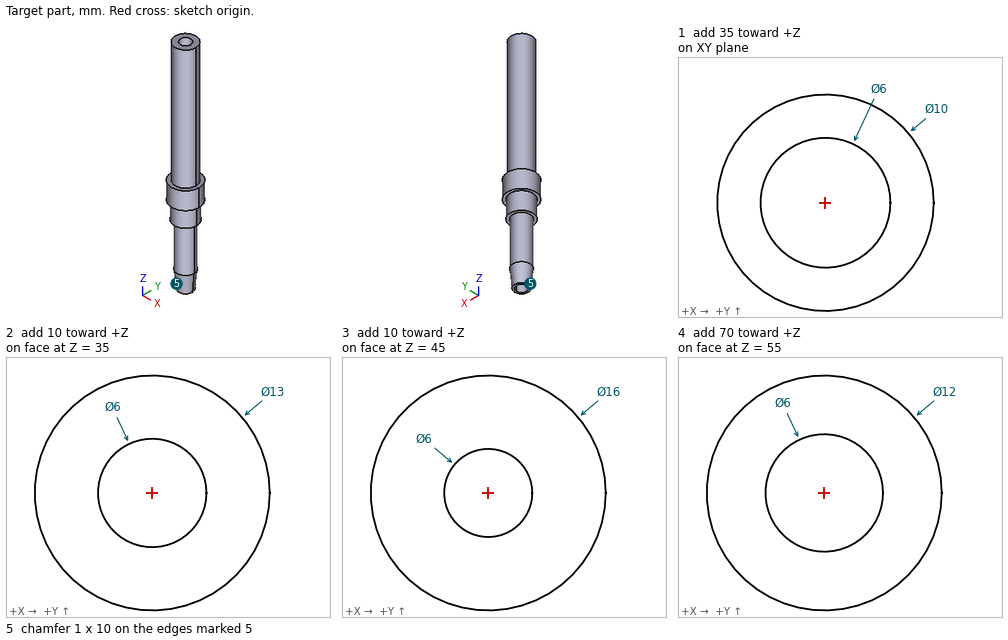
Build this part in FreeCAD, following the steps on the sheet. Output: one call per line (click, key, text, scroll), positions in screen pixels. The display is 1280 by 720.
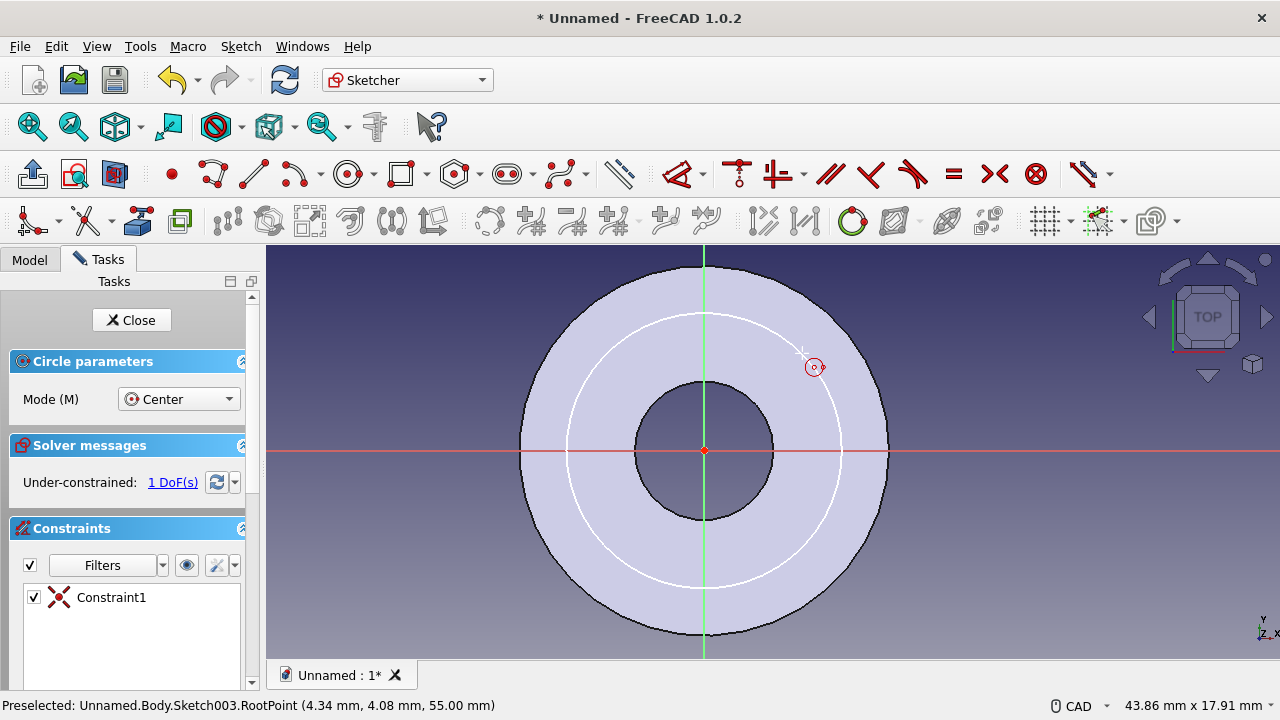
click(704, 451)
click(753, 402)
key(Escape)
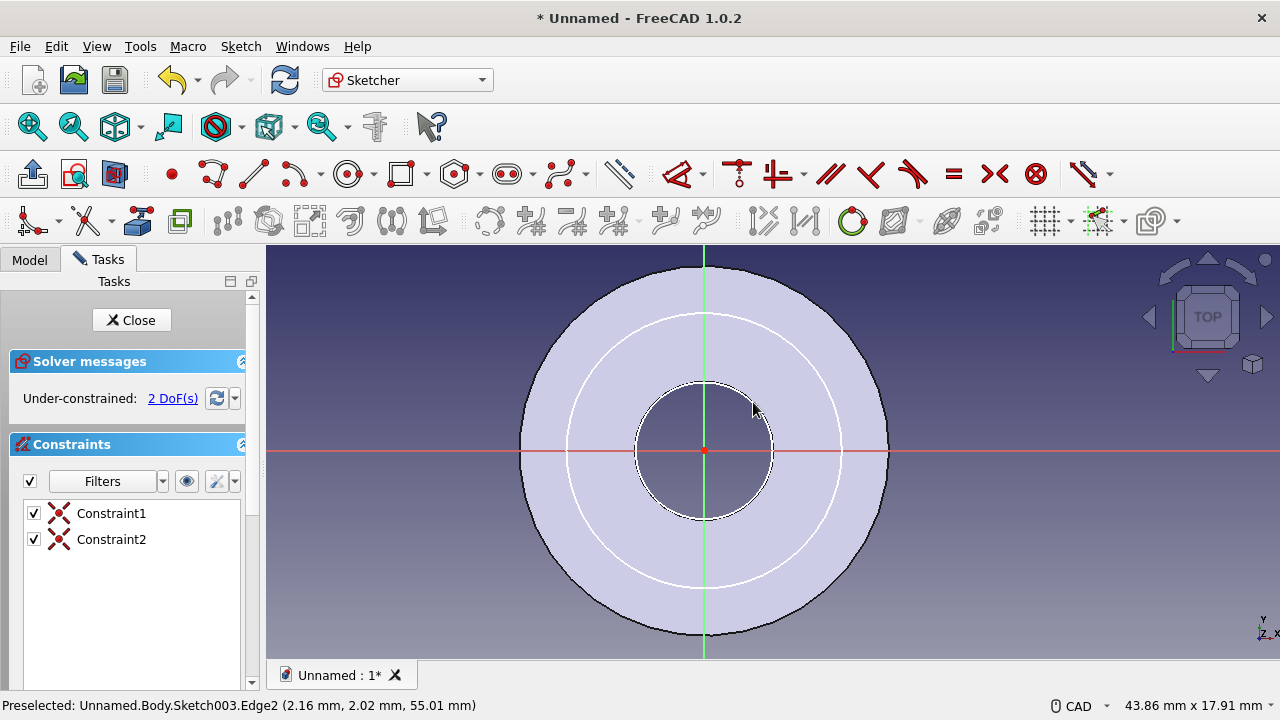
click(676, 174)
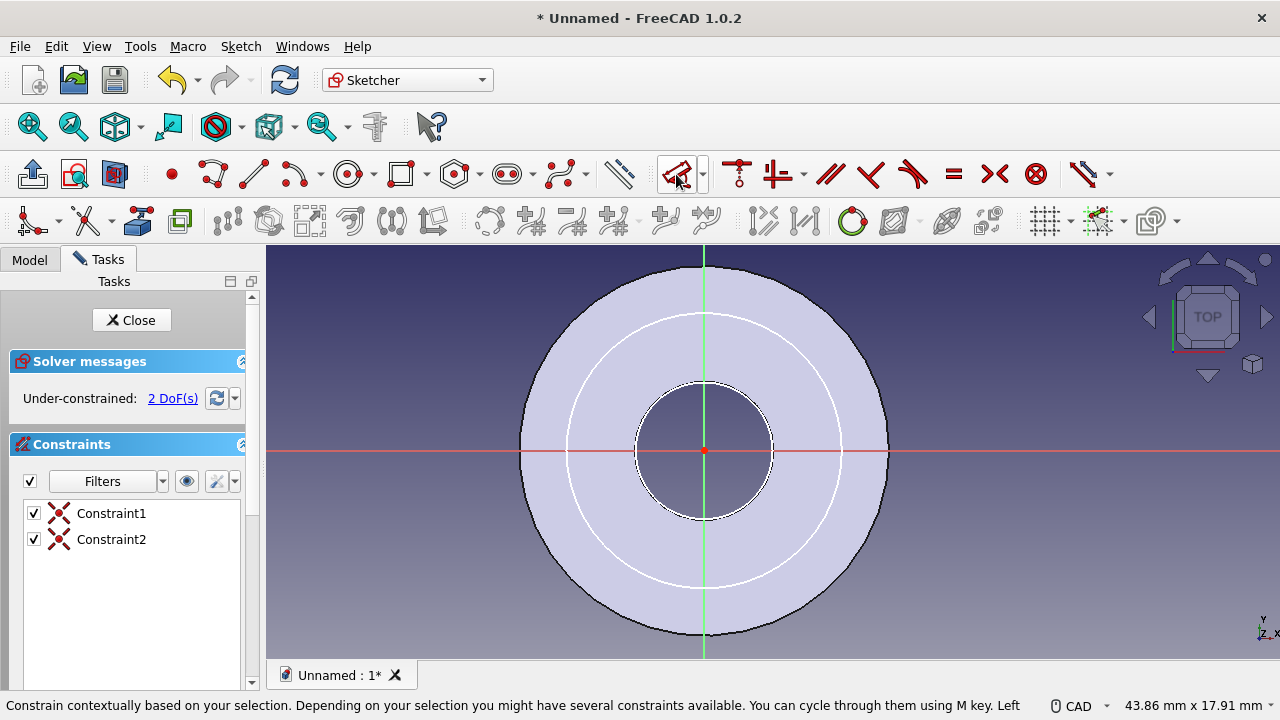
click(801, 353)
click(824, 330)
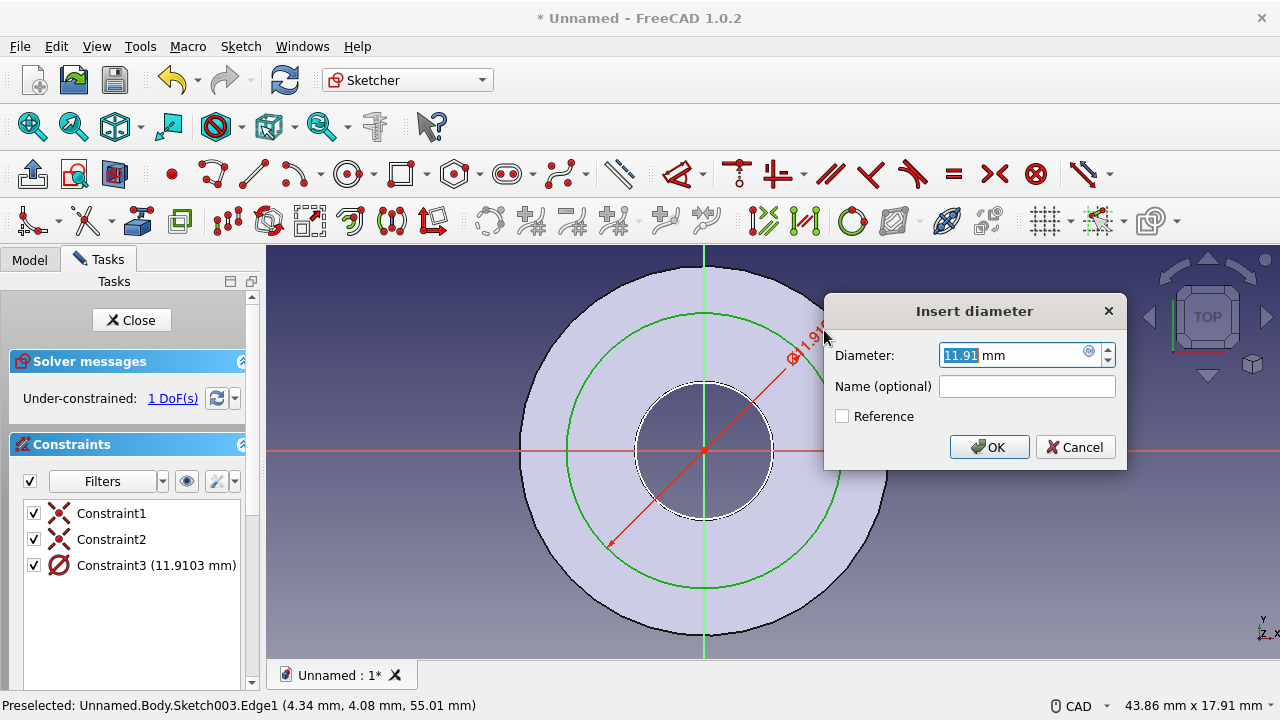
text(12)
key(Return)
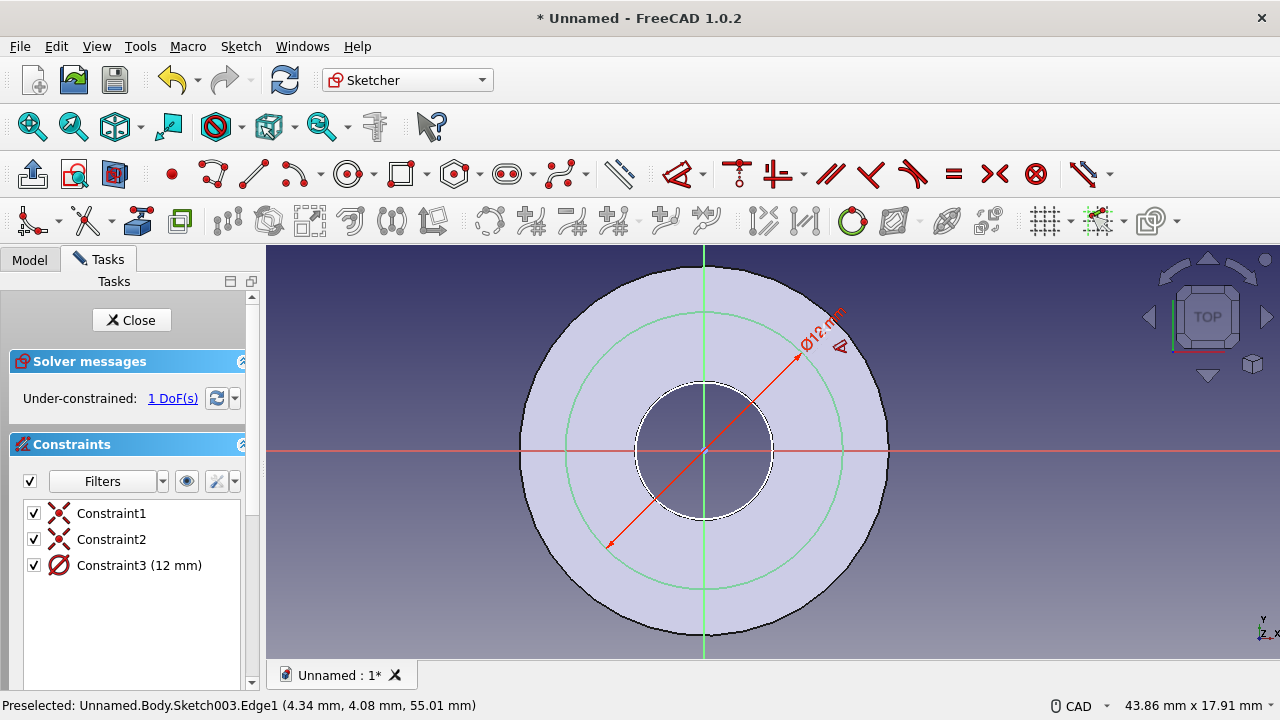
click(752, 402)
click(774, 379)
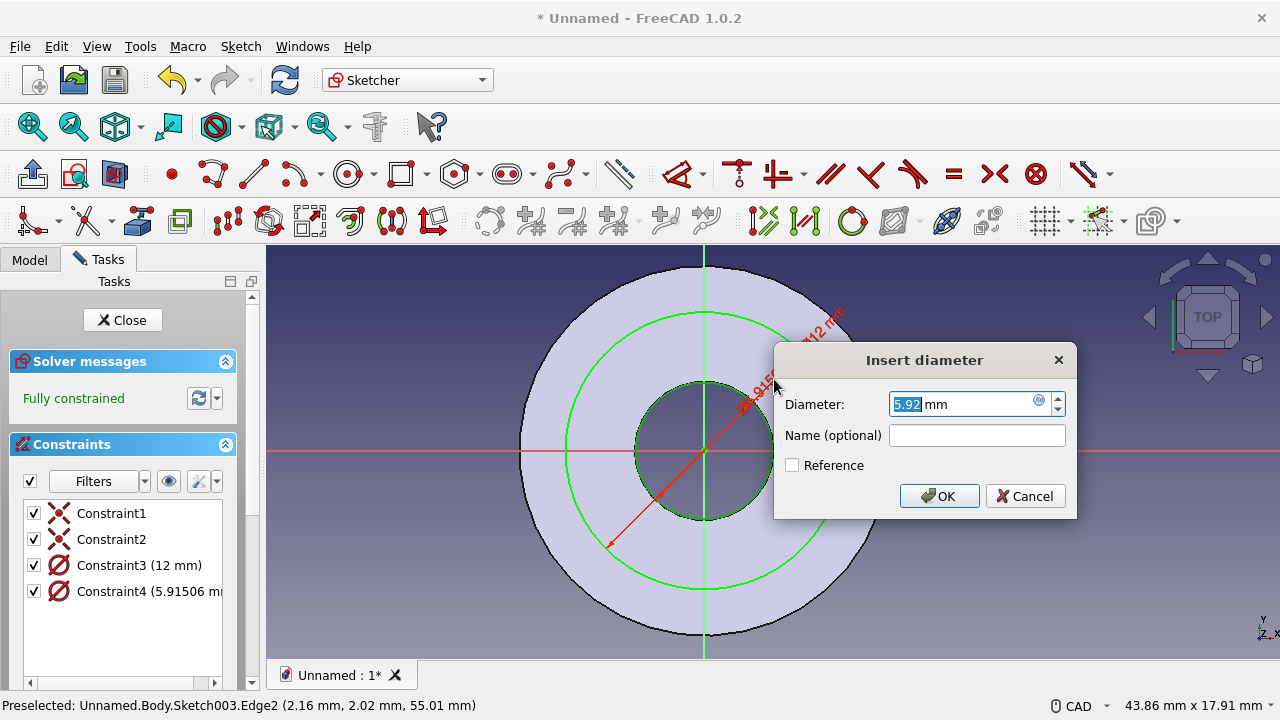
text(6)
key(Return)
key(Escape)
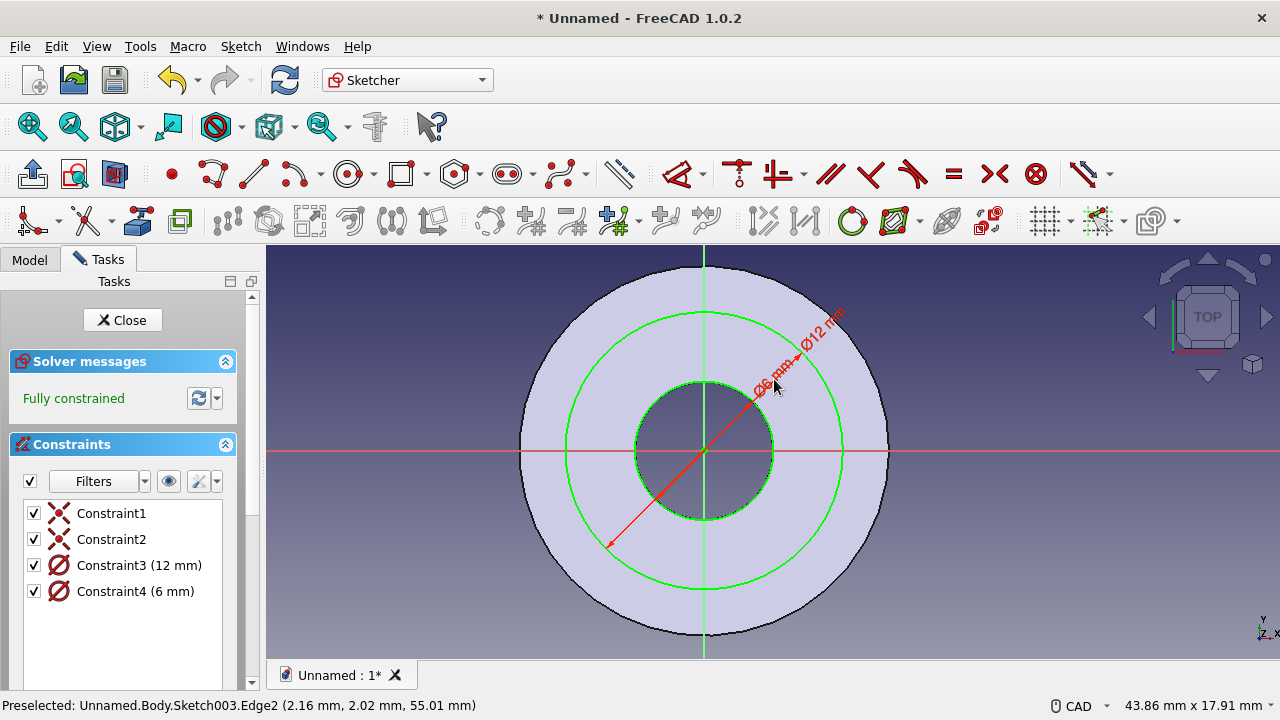
click(123, 320)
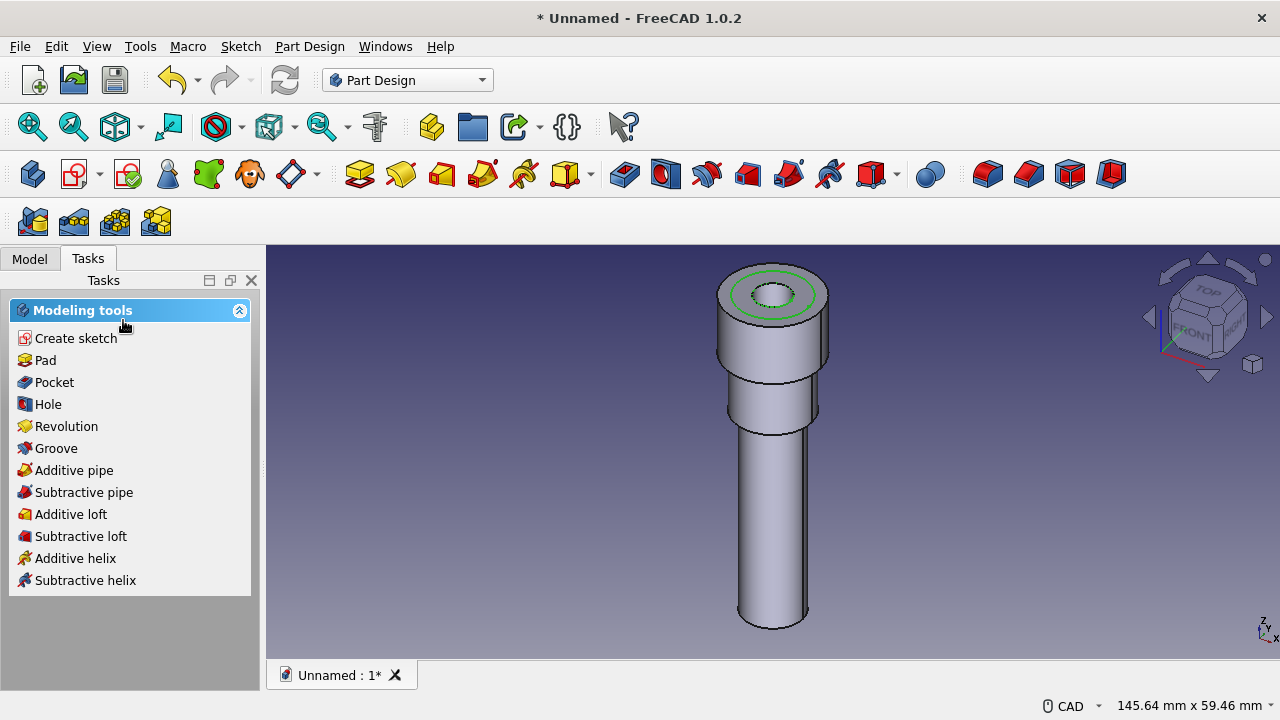
click(360, 174)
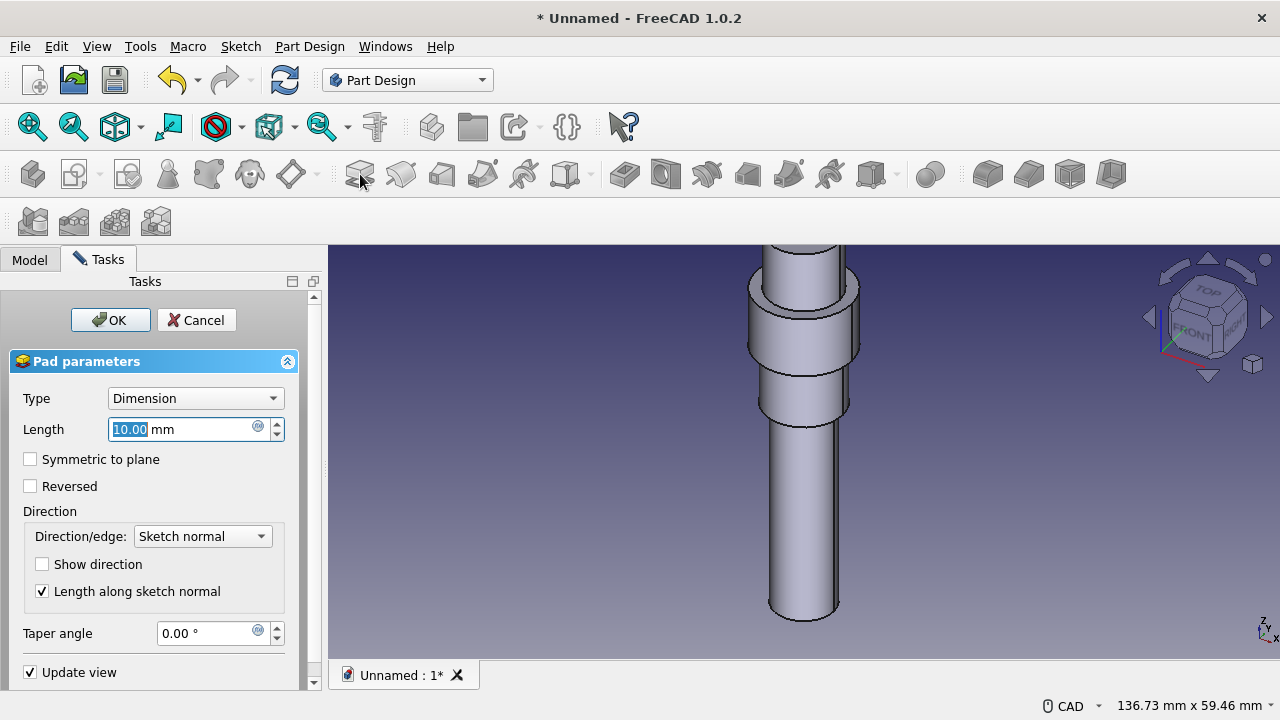
text(70)
key(Tab)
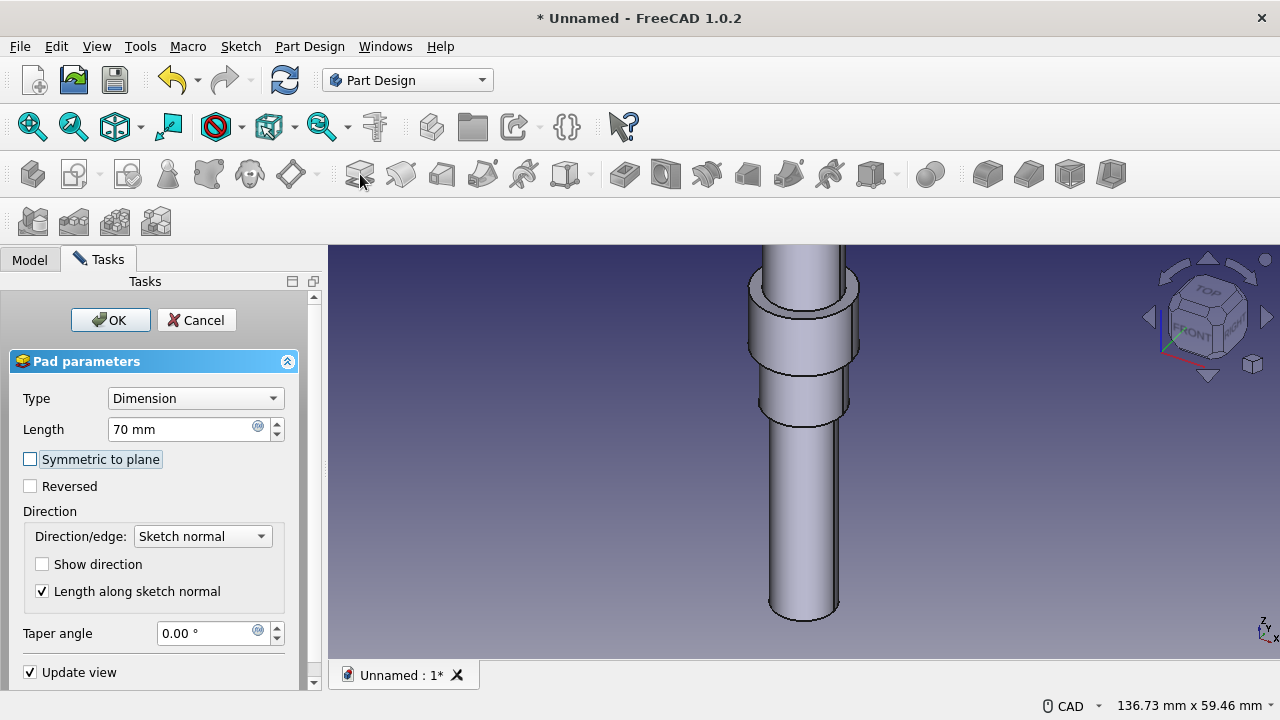
click(111, 320)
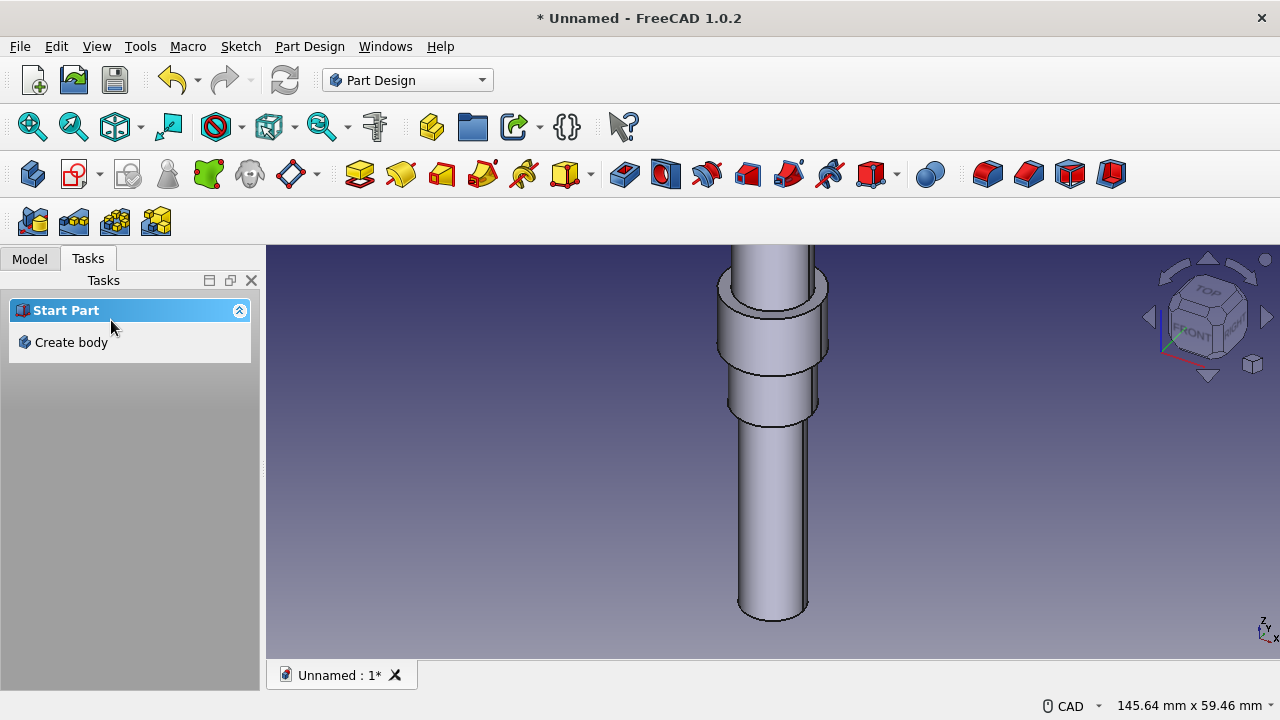
click(33, 128)